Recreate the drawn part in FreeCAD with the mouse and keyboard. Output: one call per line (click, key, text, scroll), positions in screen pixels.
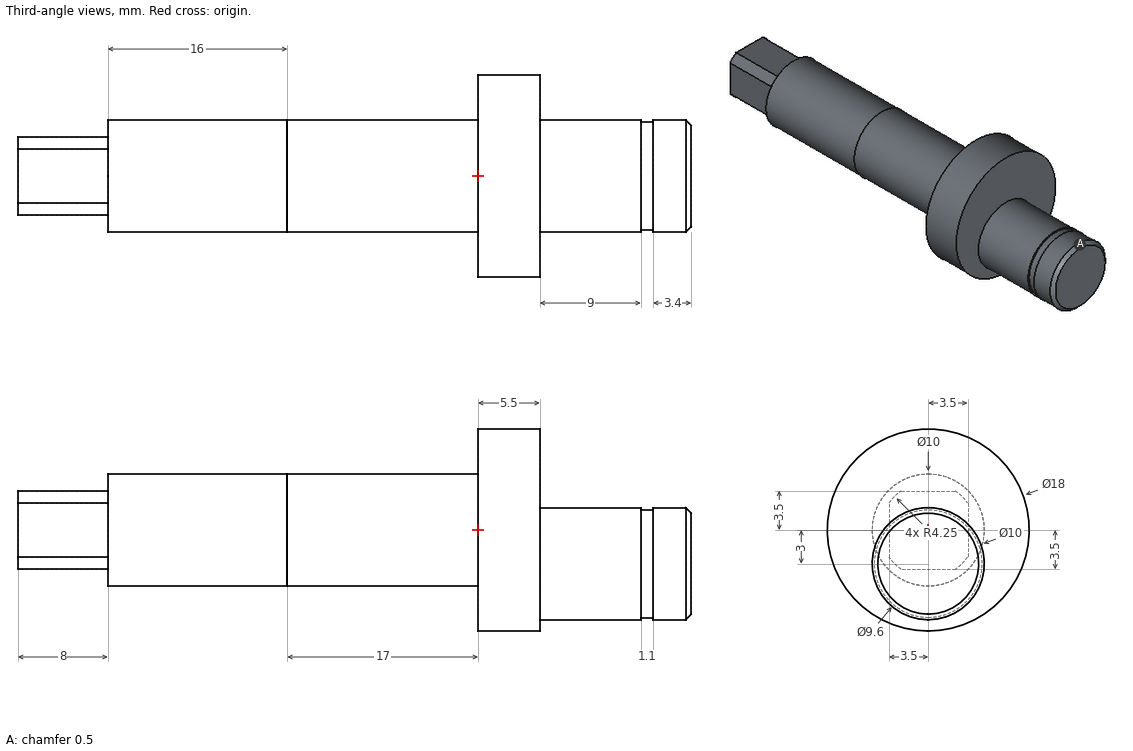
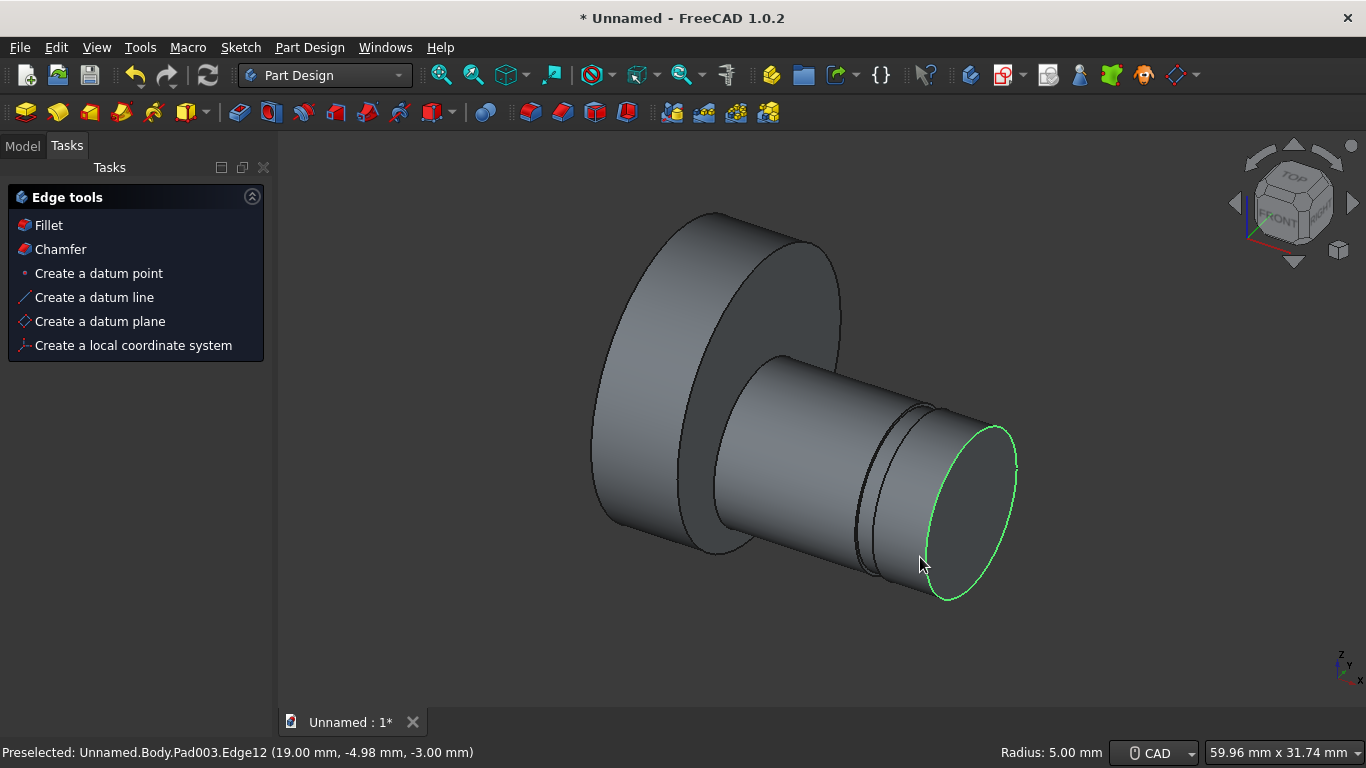
click(564, 112)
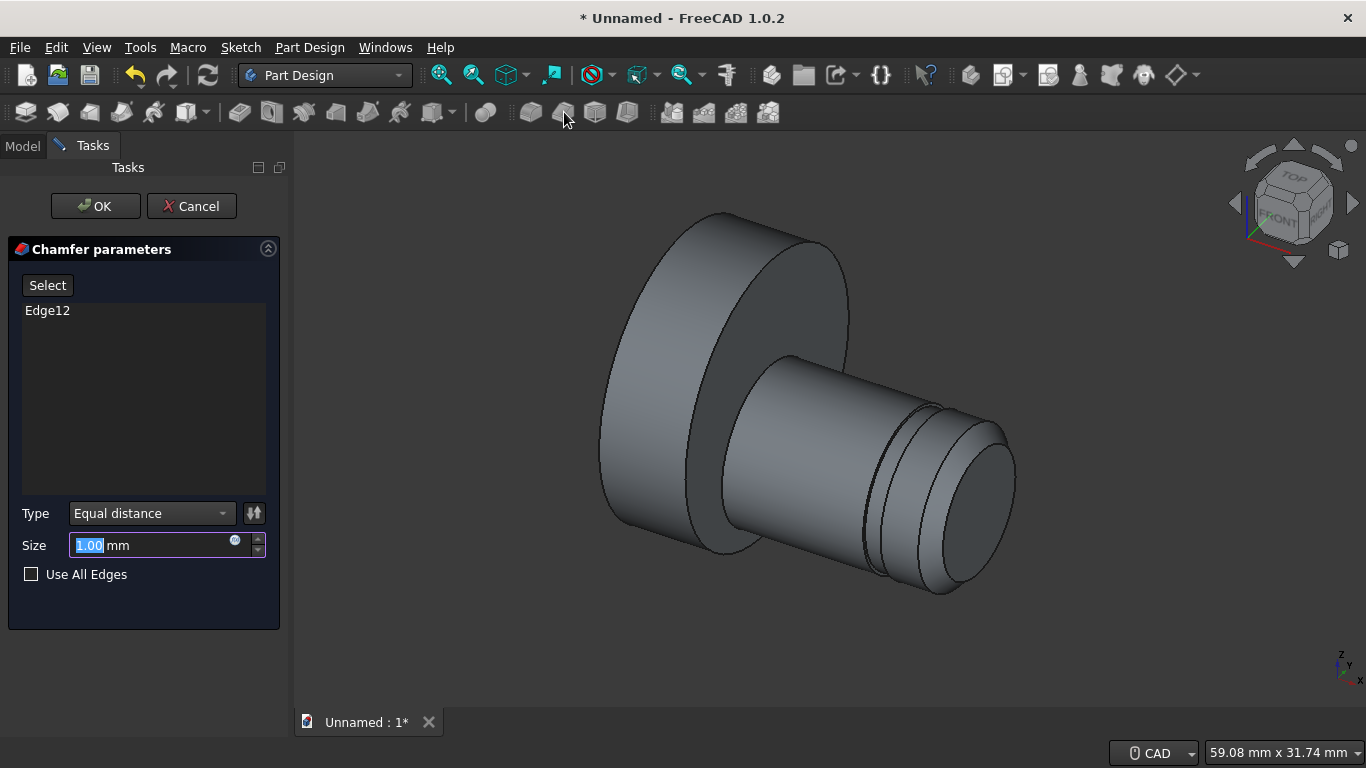
text(0.5)
key(Tab)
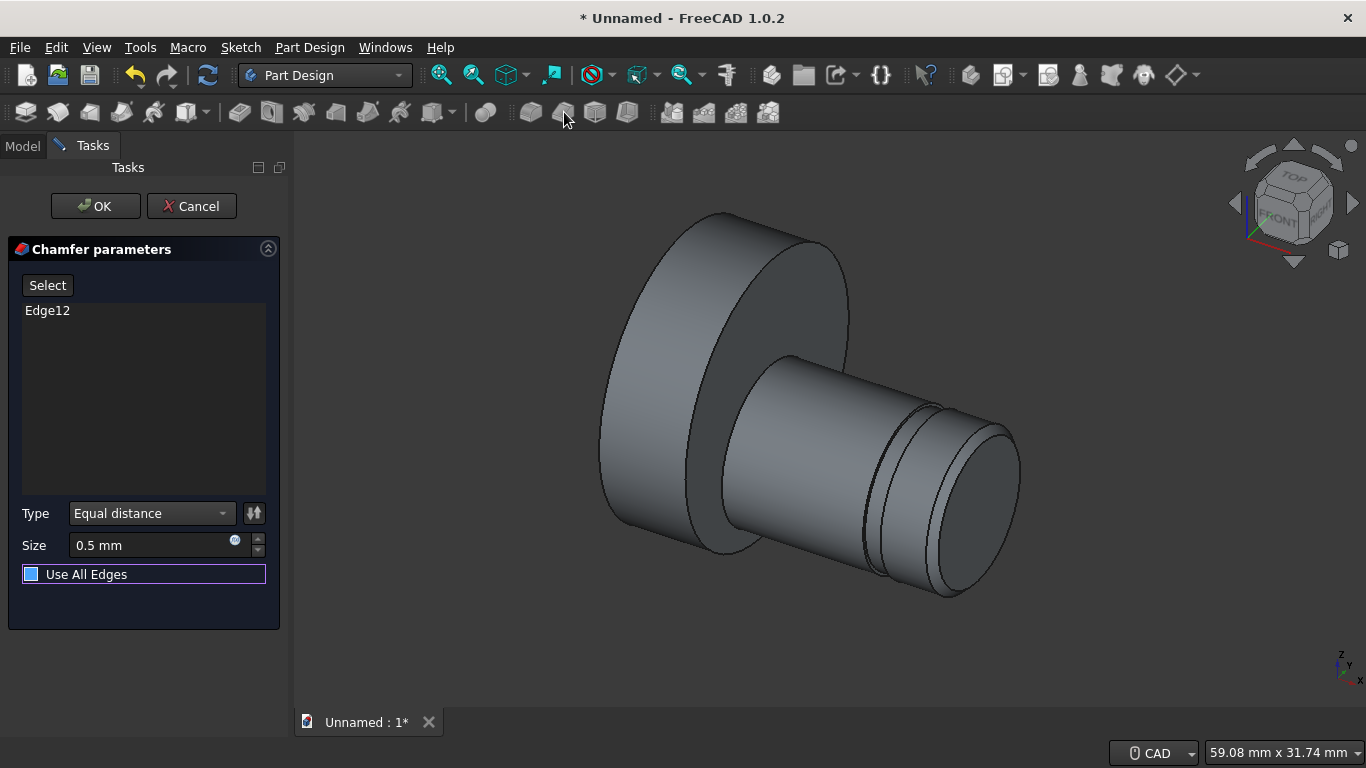
click(96, 206)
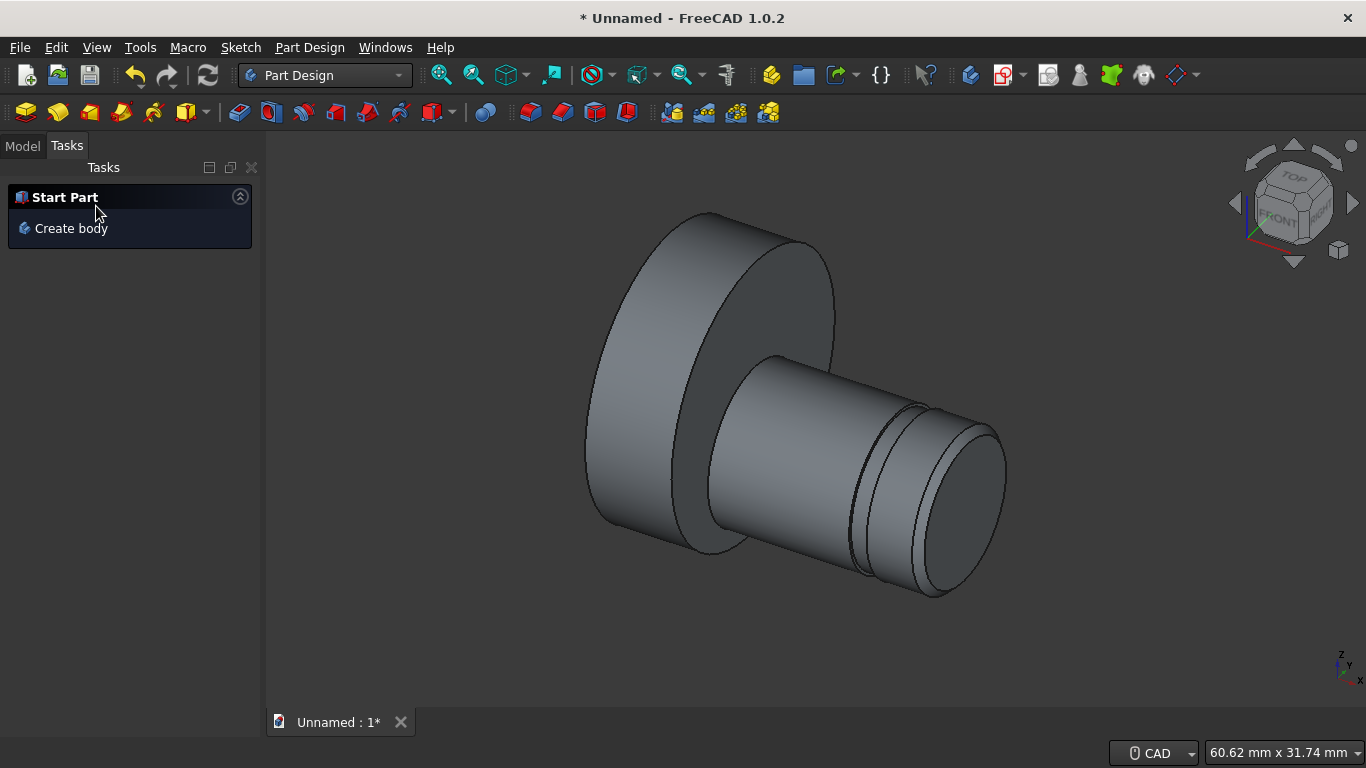
key(6)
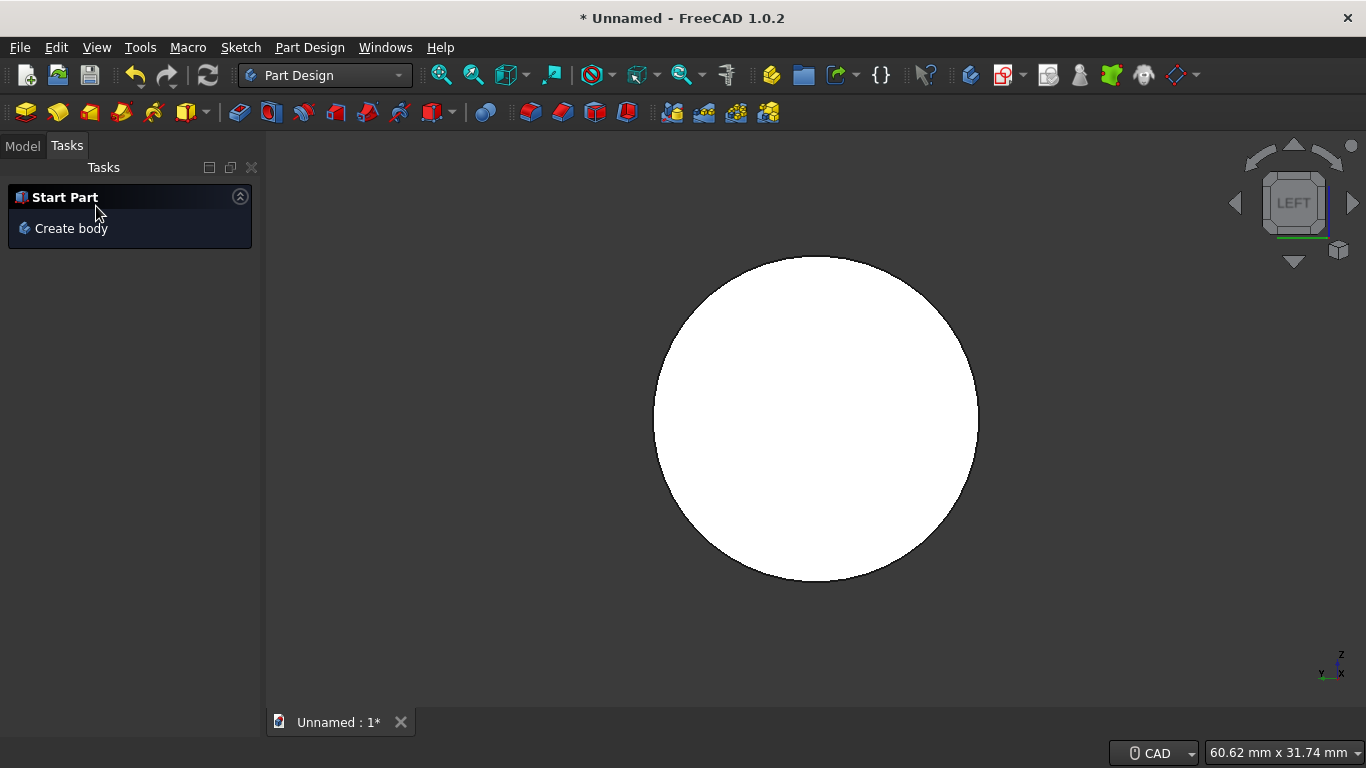
click(816, 418)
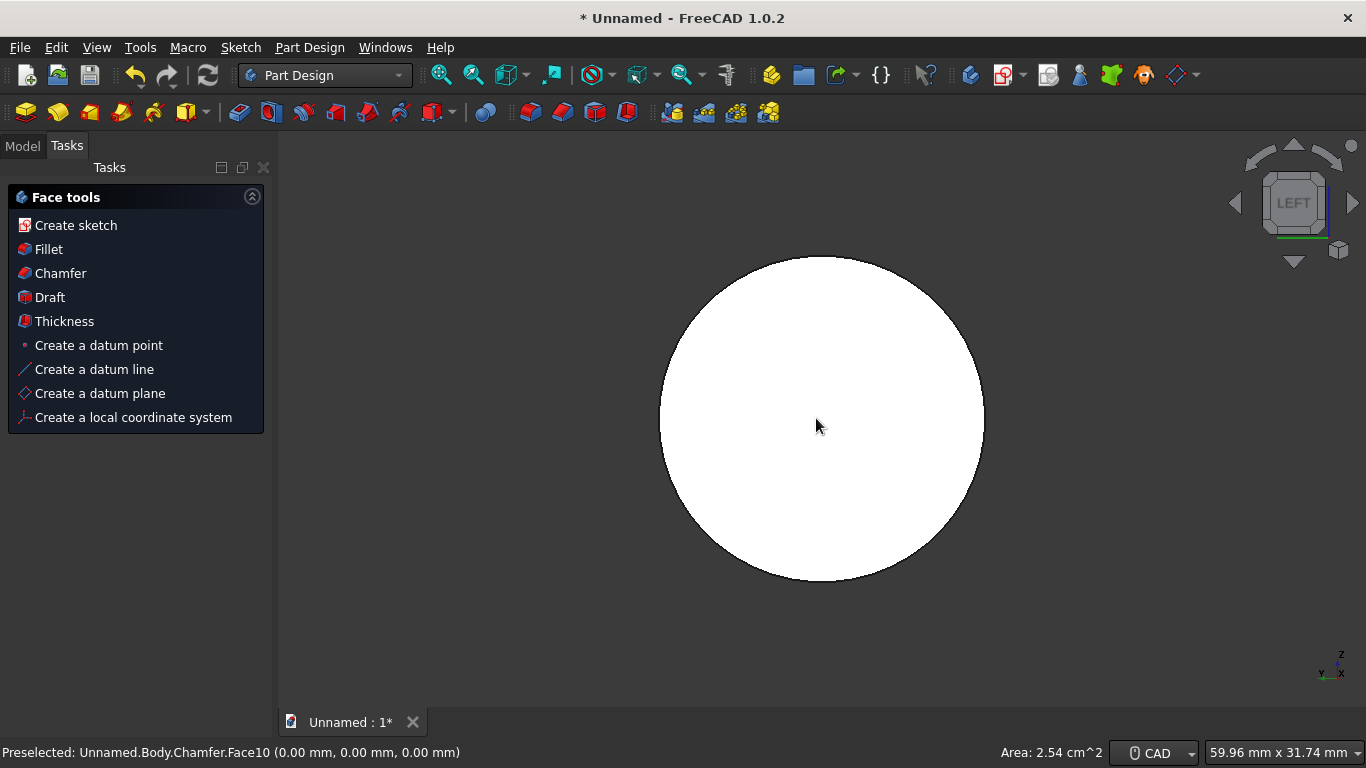
click(1004, 76)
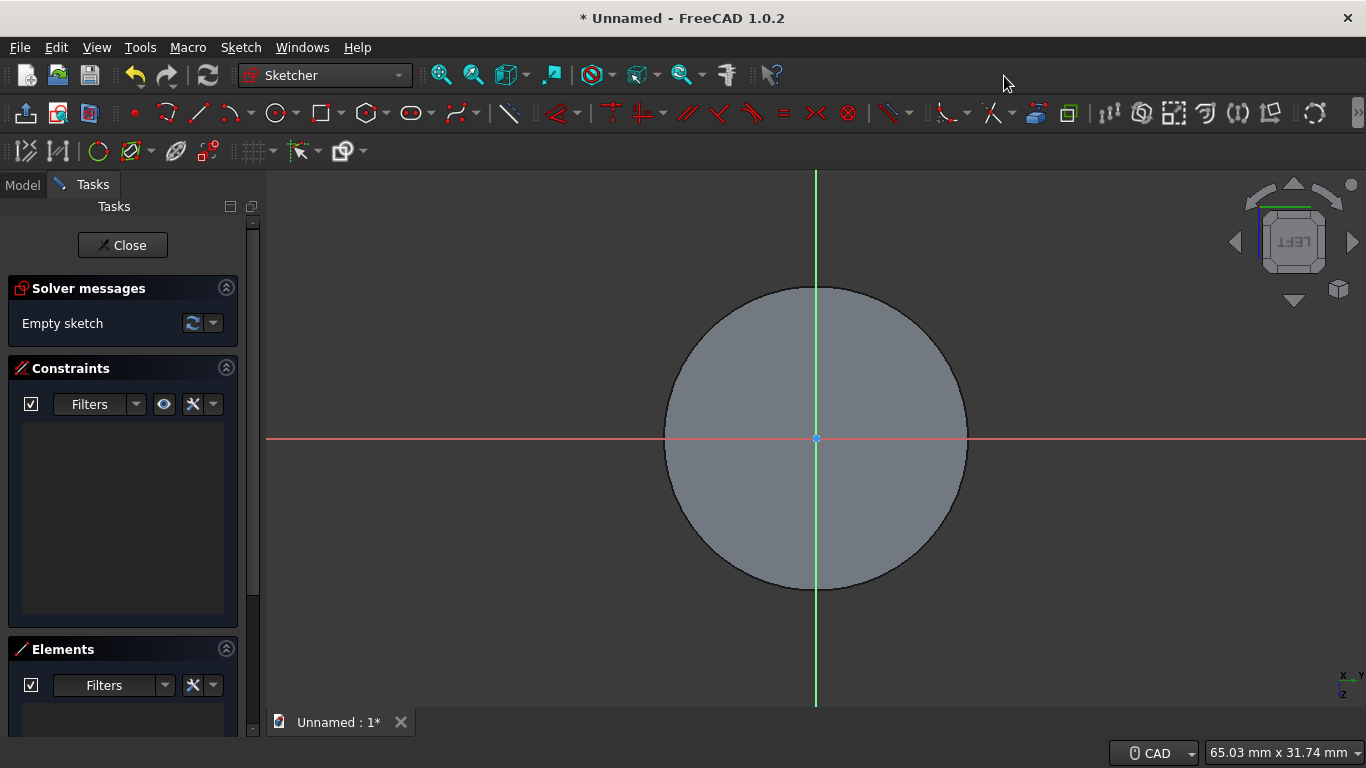
scroll(899, 438, up, 3)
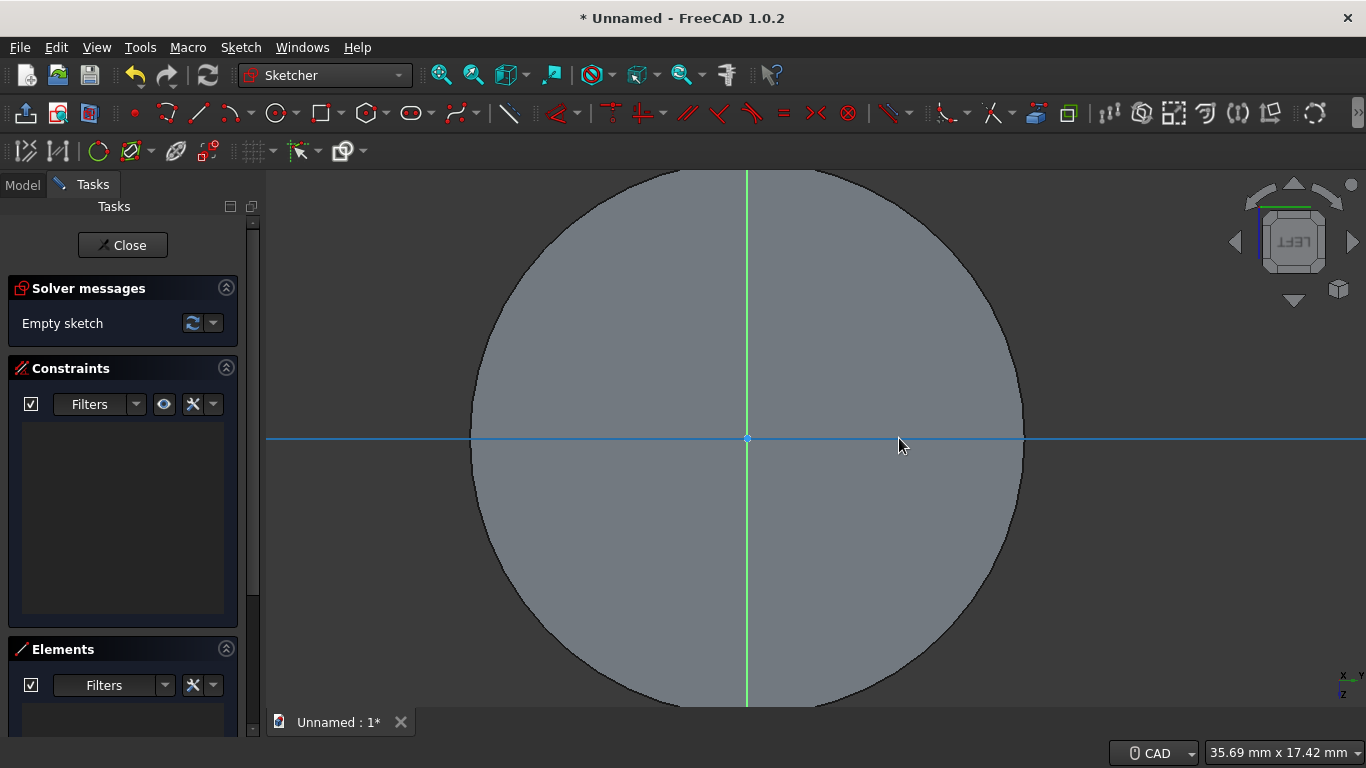
key(g)
key(c)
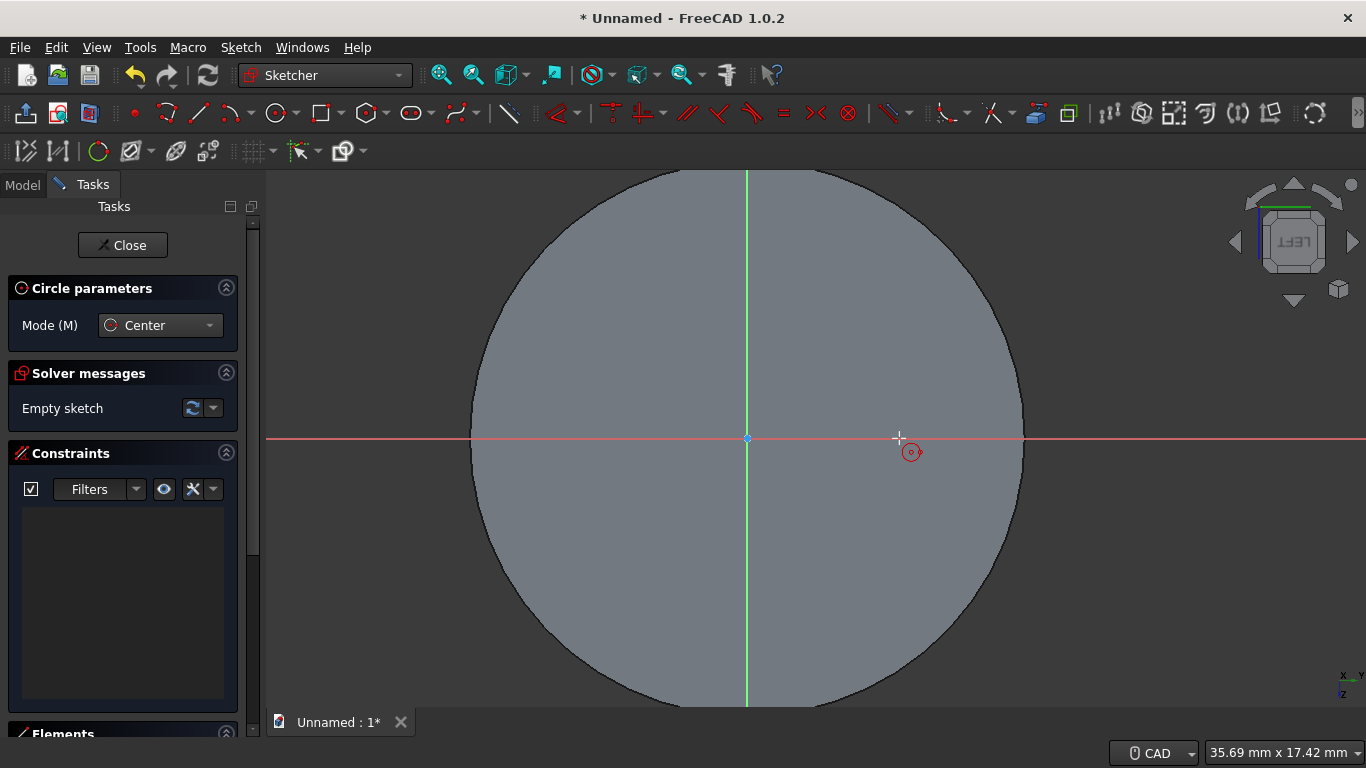
click(747, 438)
click(856, 330)
key(Escape)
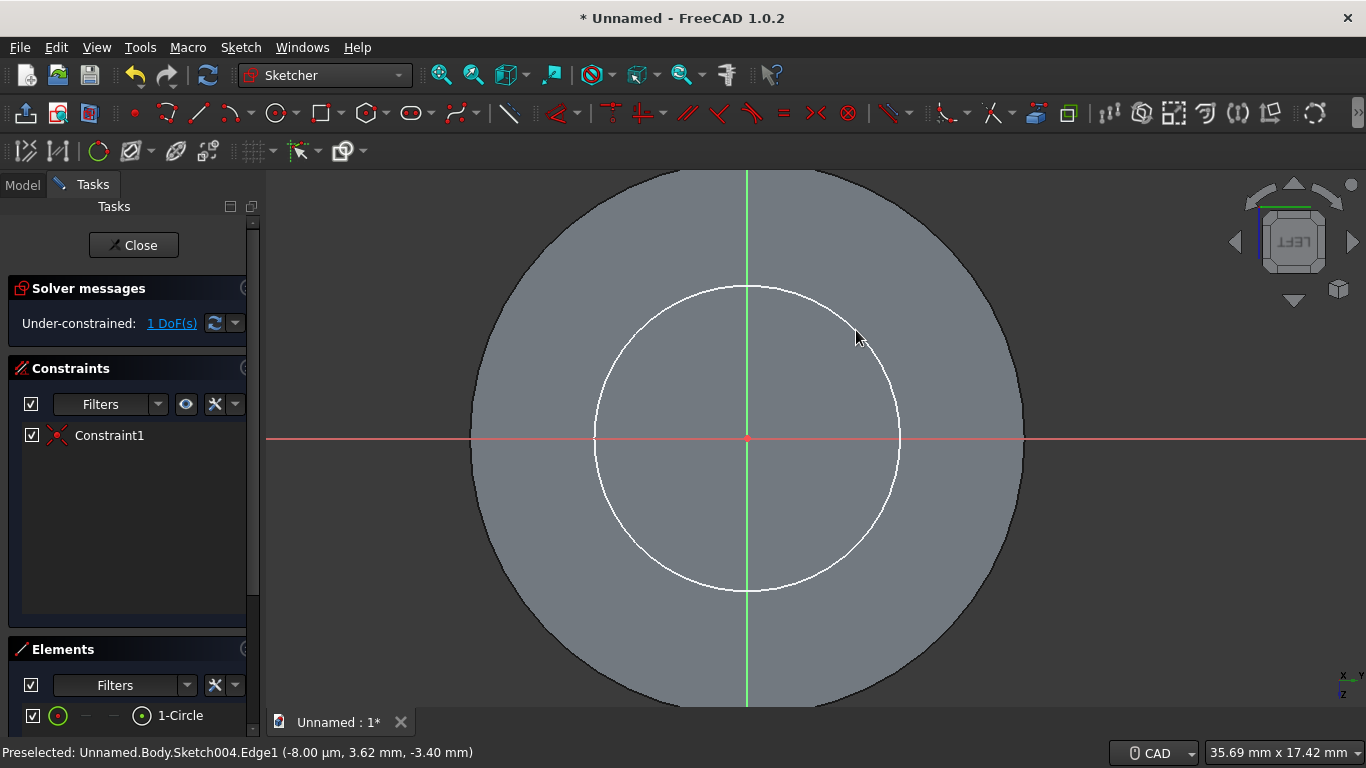
key(d)